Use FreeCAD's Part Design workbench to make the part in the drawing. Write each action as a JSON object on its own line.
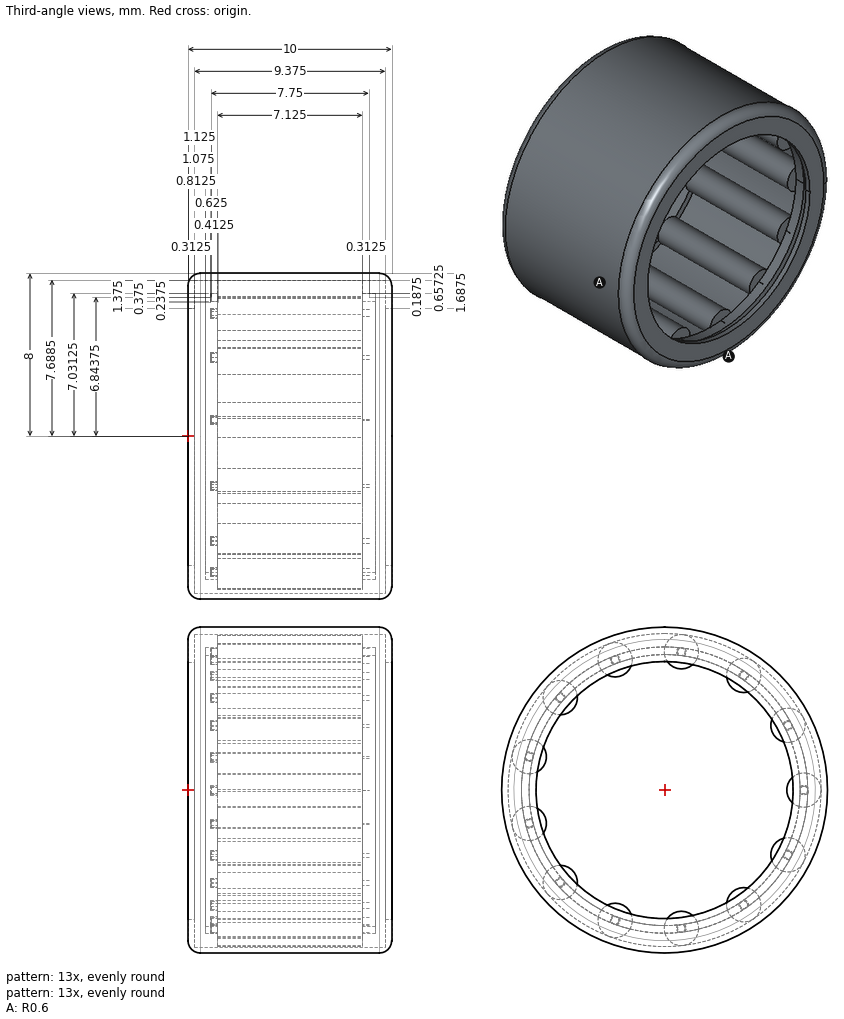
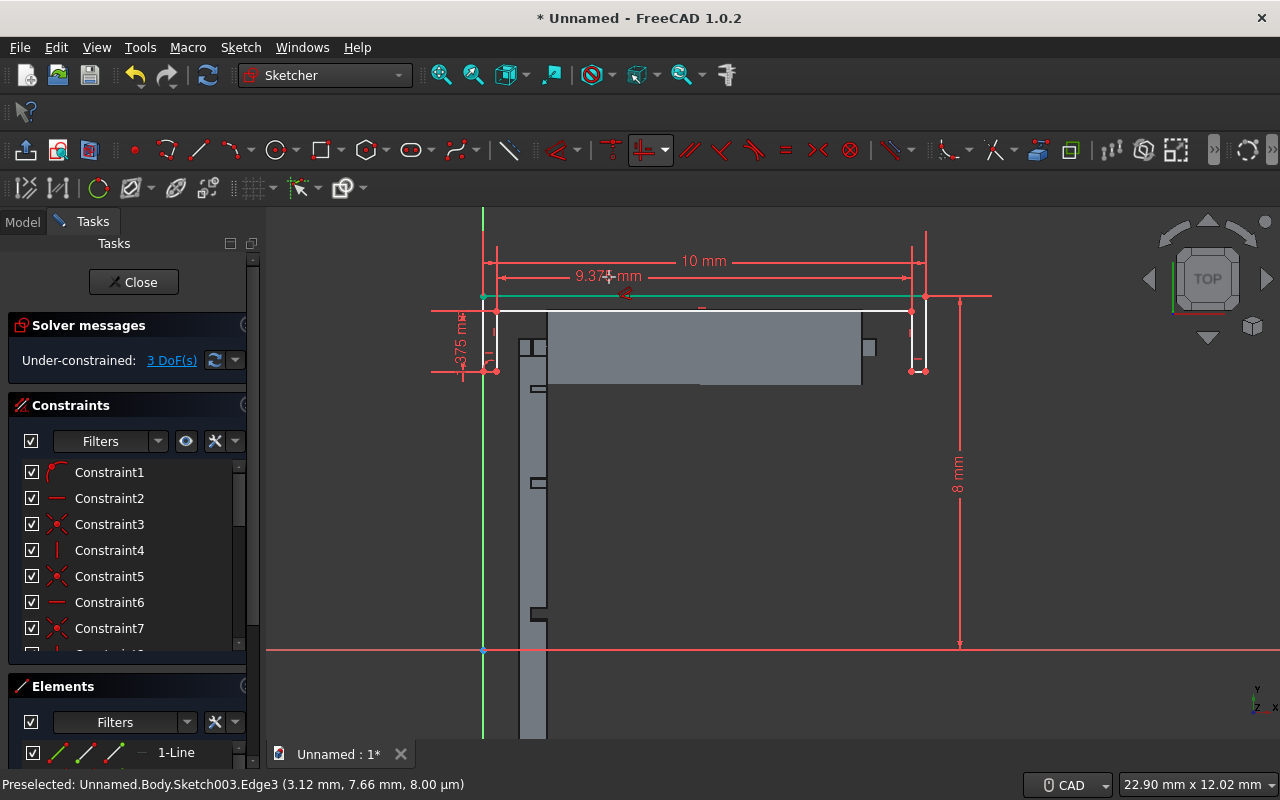
{"action": "left_click", "coordinate": [912, 329]}
{"action": "left_click", "coordinate": [946, 342]}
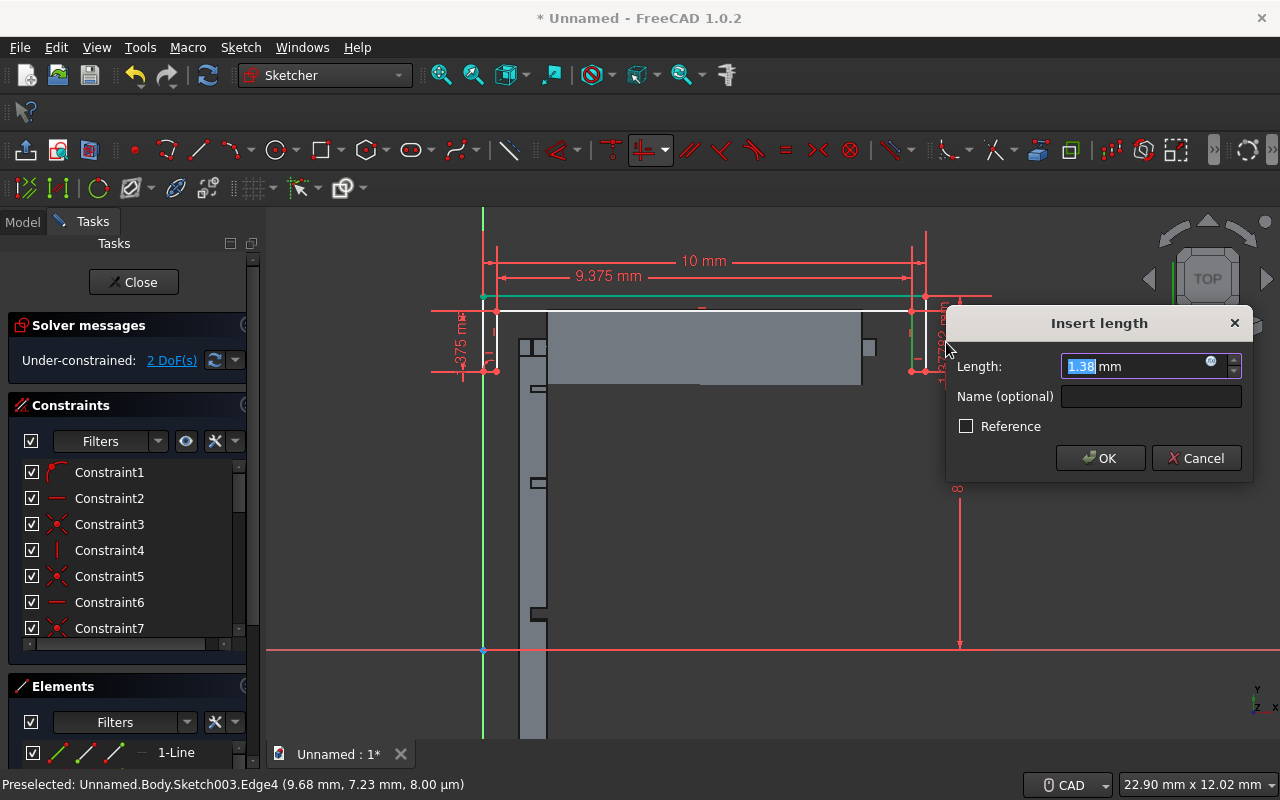
{"action": "type", "text": "1.375"}
{"action": "key", "text": "Return"}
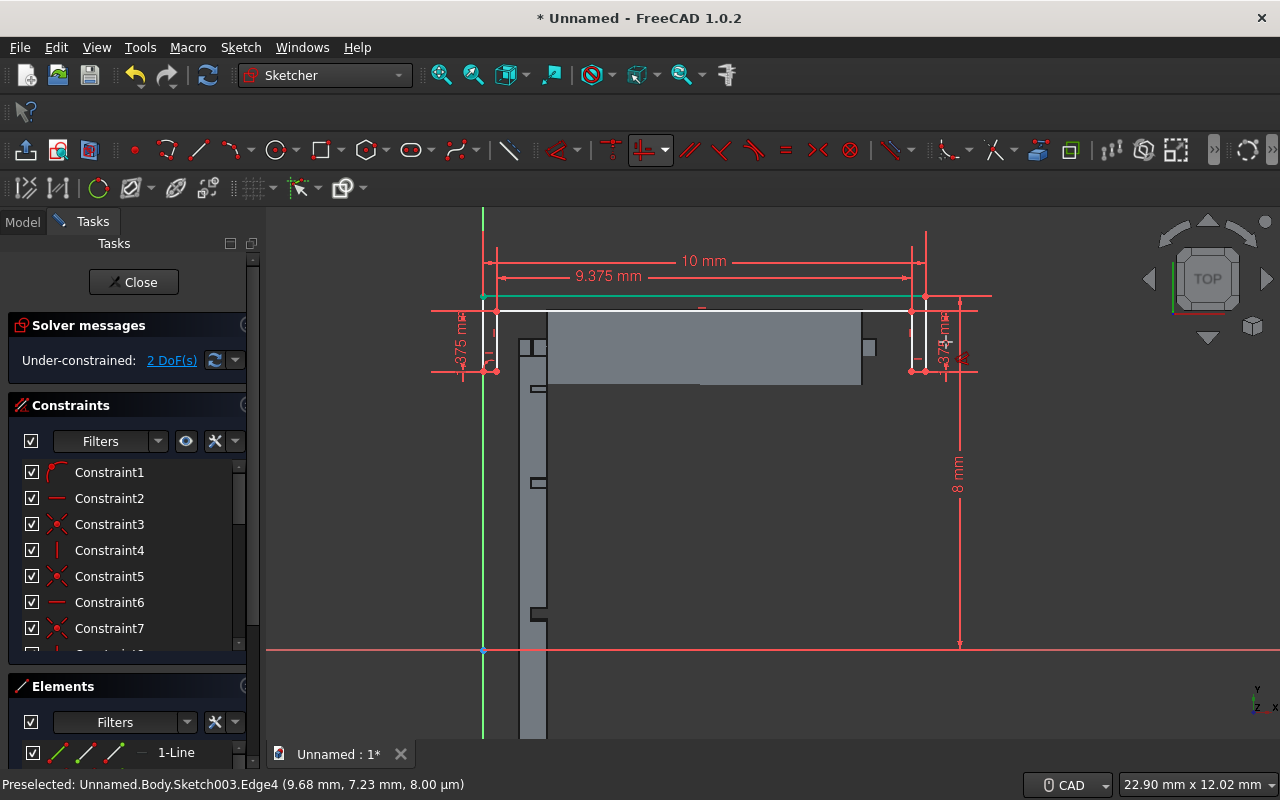
{"action": "scroll", "coordinate": [490, 372], "scroll_direction": "up", "scroll_amount": 6}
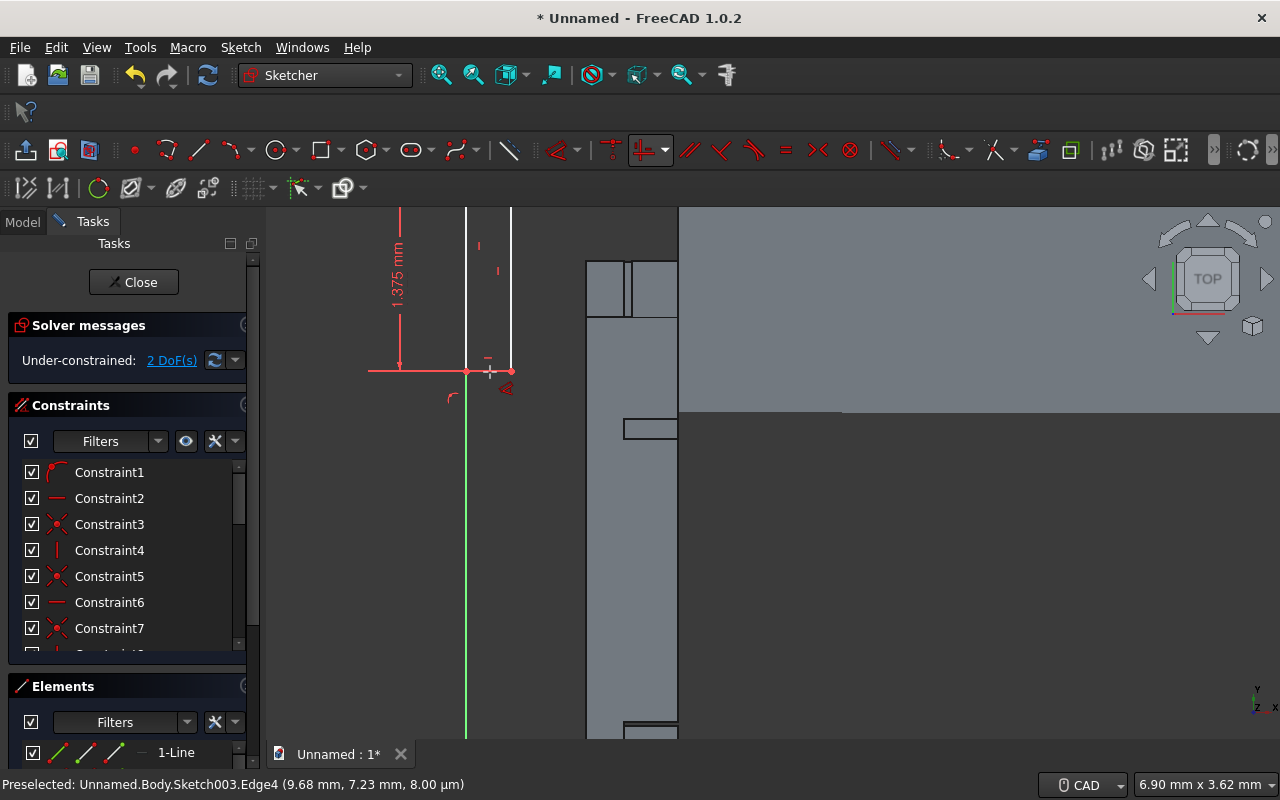
{"action": "left_click", "coordinate": [489, 371]}
{"action": "left_click", "coordinate": [489, 337]}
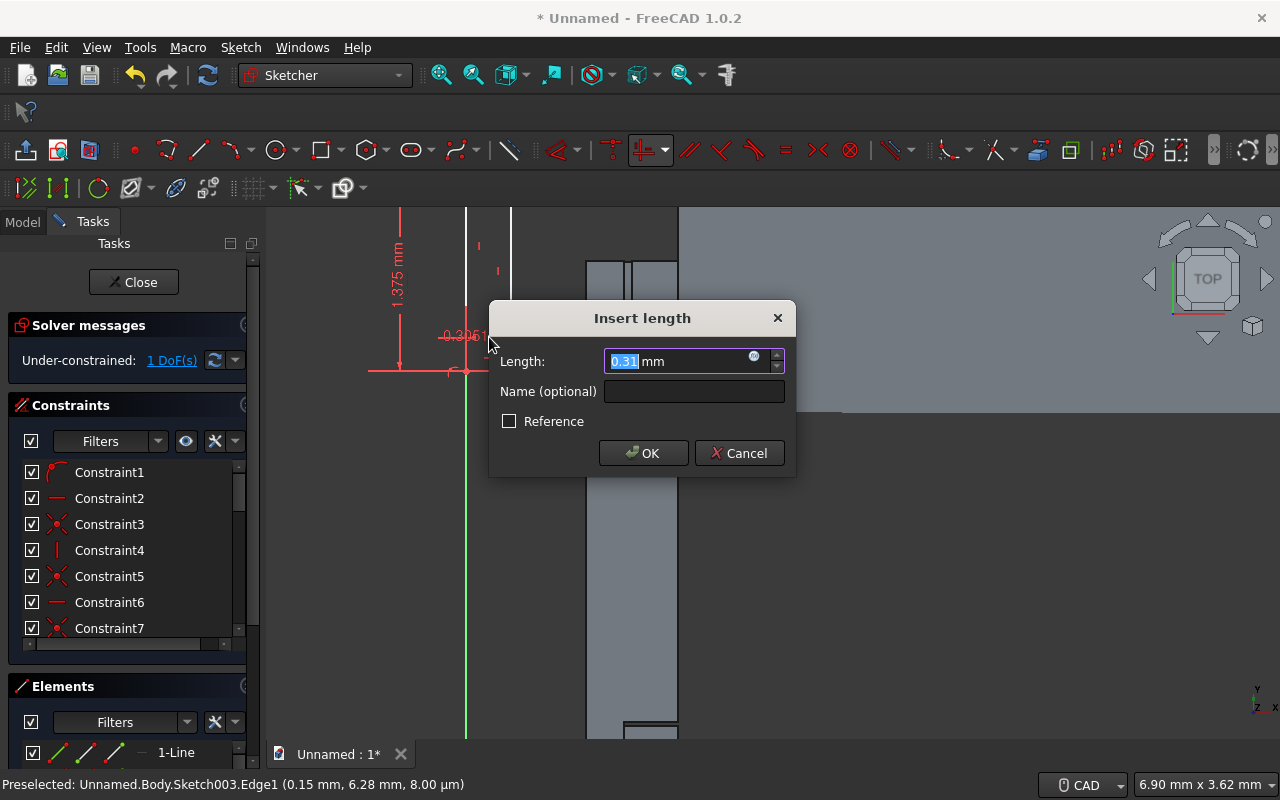
{"action": "type", "text": "0.3125"}
{"action": "key", "text": "Return"}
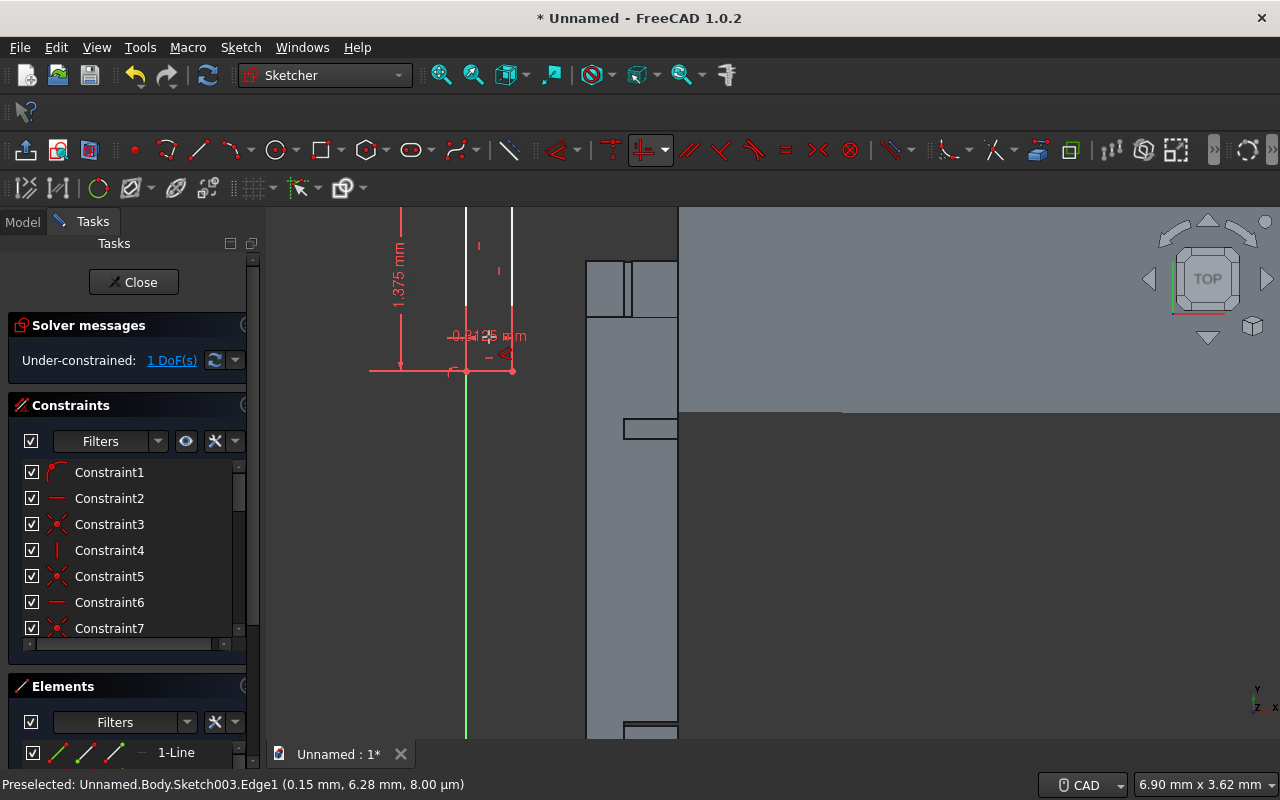
{"action": "scroll", "coordinate": [490, 372], "scroll_direction": "down", "scroll_amount": 6}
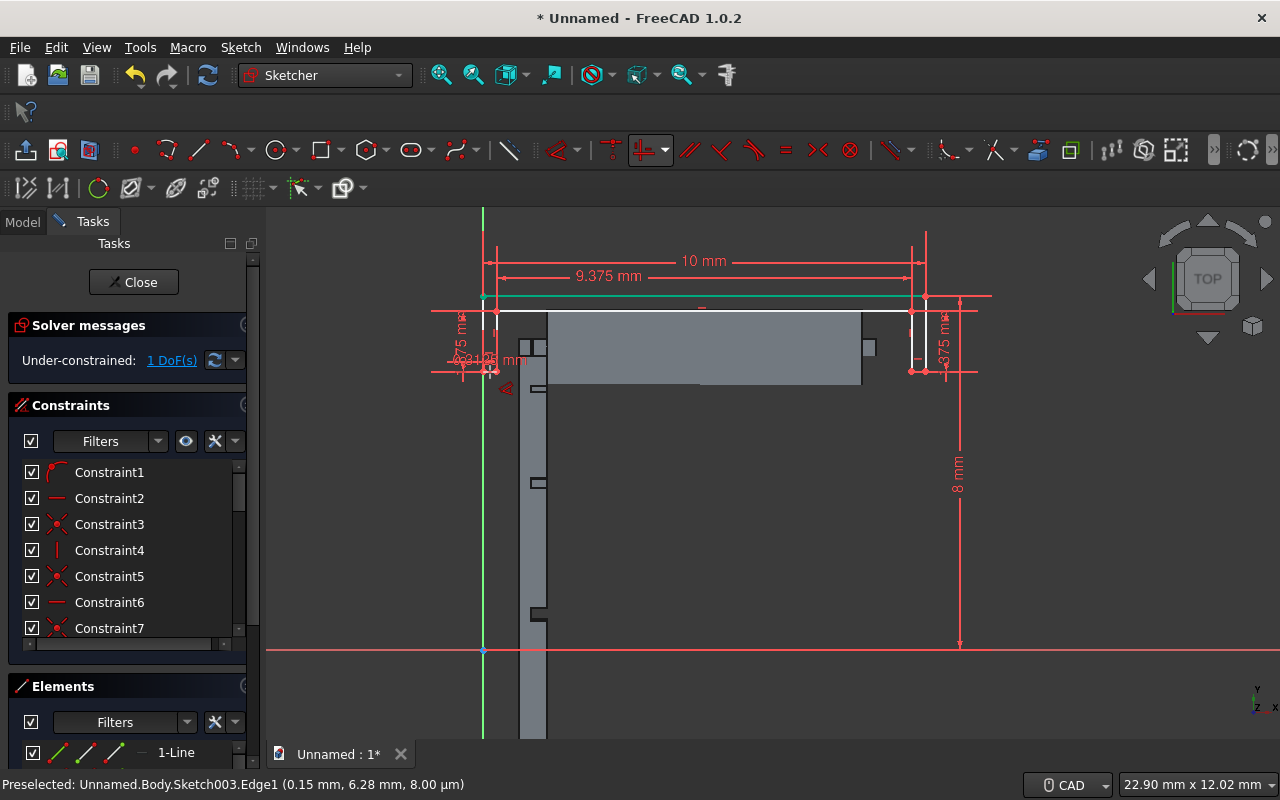
{"action": "left_click", "coordinate": [926, 349]}
{"action": "left_click", "coordinate": [960, 317]}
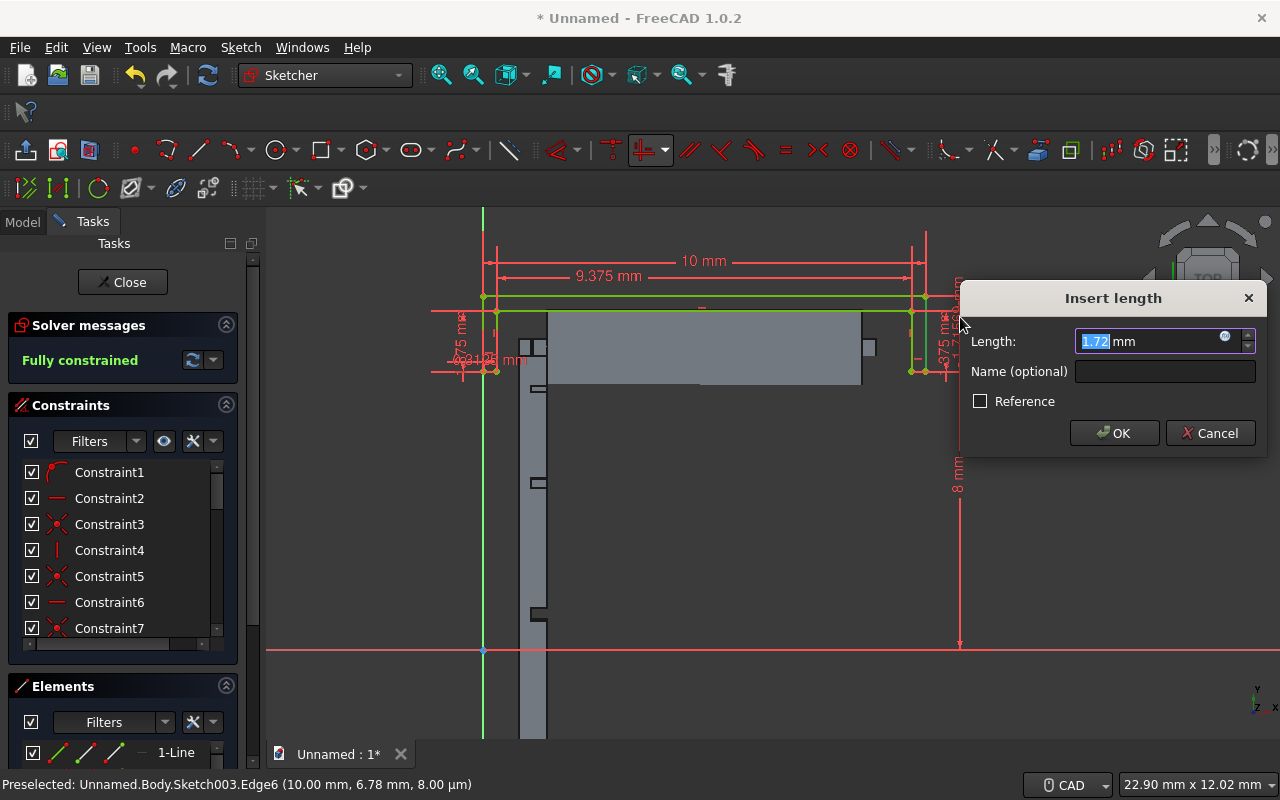
{"action": "type", "text": "1.6875"}
{"action": "key", "text": "Return"}
{"action": "key", "text": "Escape"}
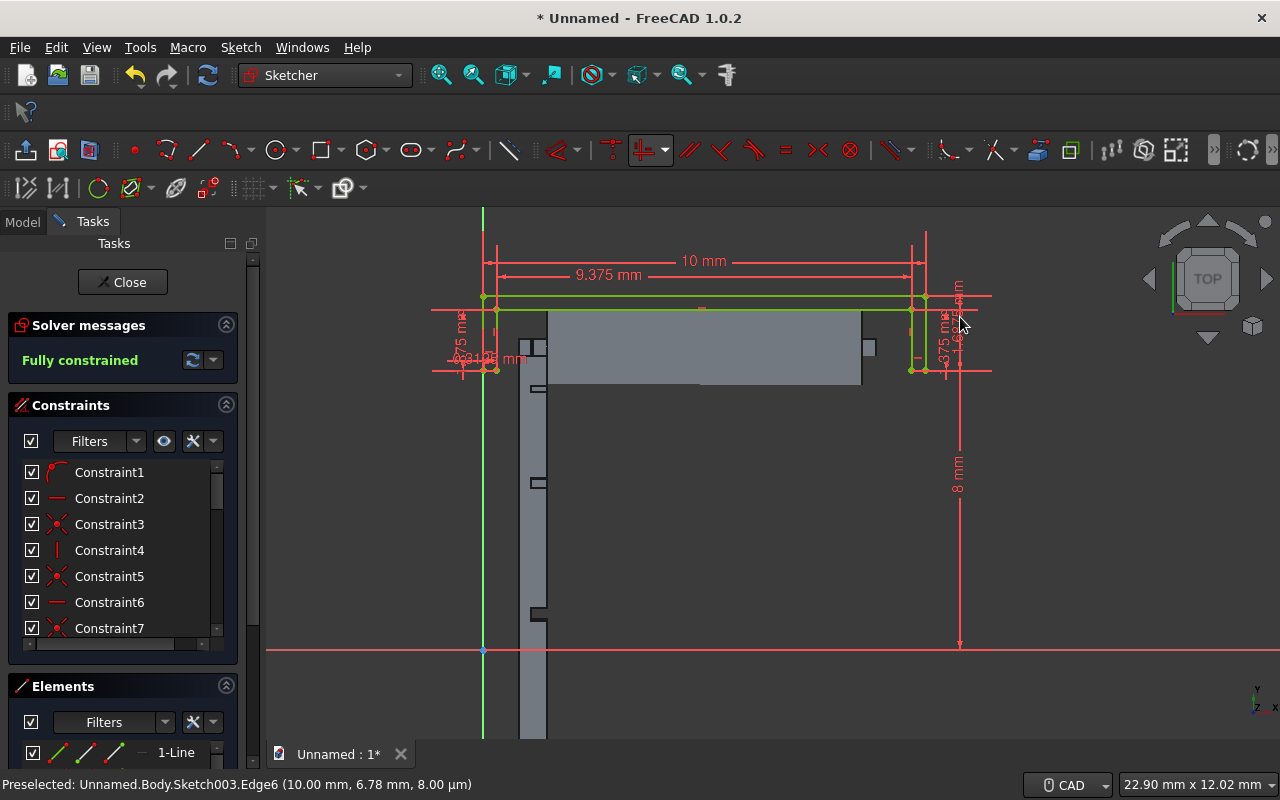
{"action": "left_click", "coordinate": [123, 282]}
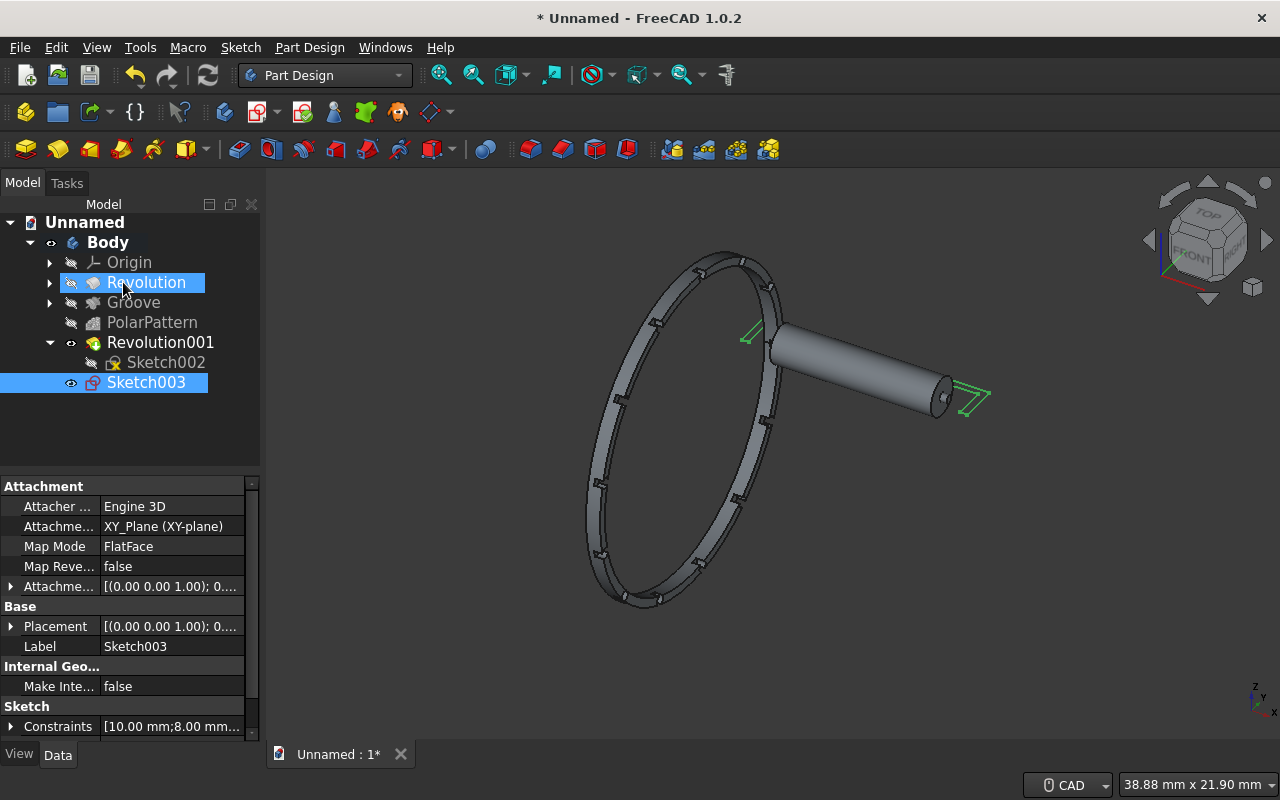
{"action": "left_click", "coordinate": [58, 150]}